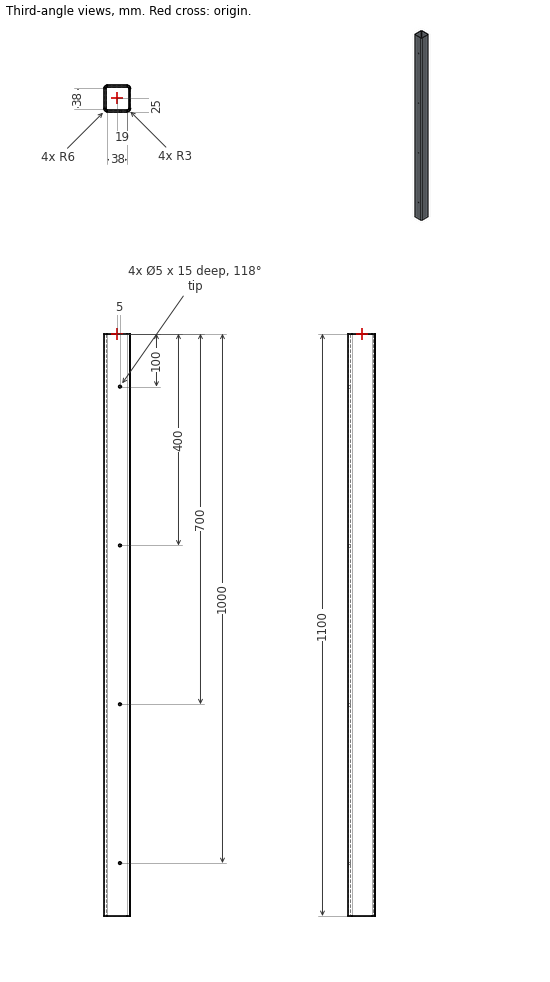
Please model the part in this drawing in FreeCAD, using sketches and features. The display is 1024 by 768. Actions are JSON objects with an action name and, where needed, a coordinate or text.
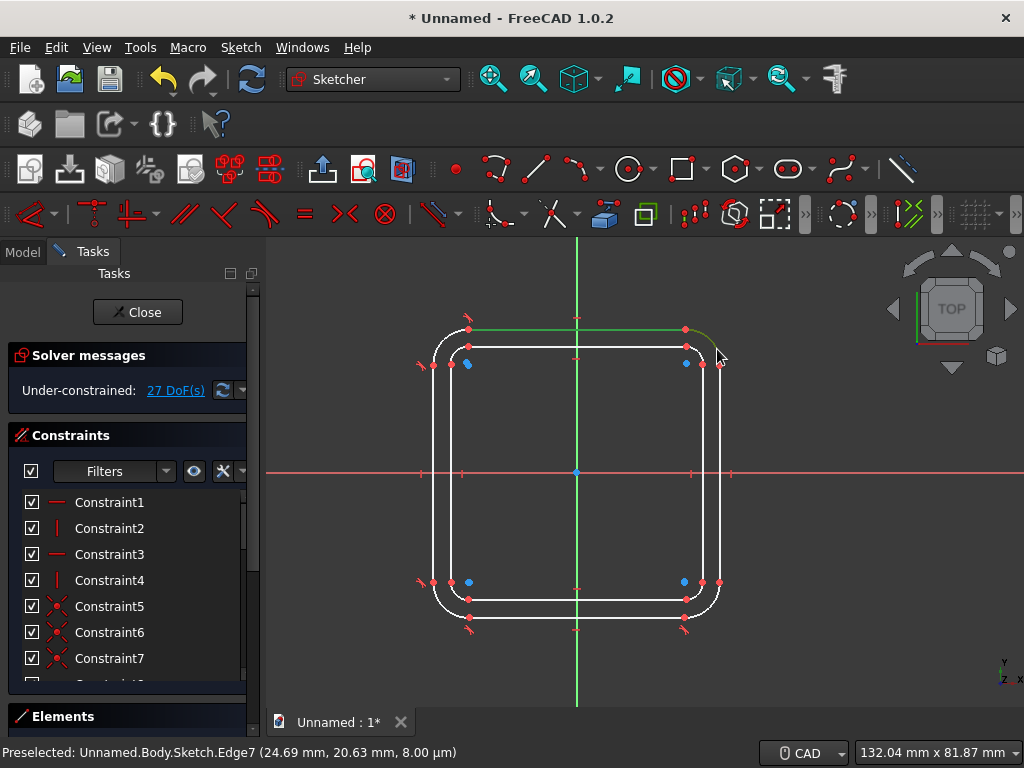
{"action": "key", "text": "t"}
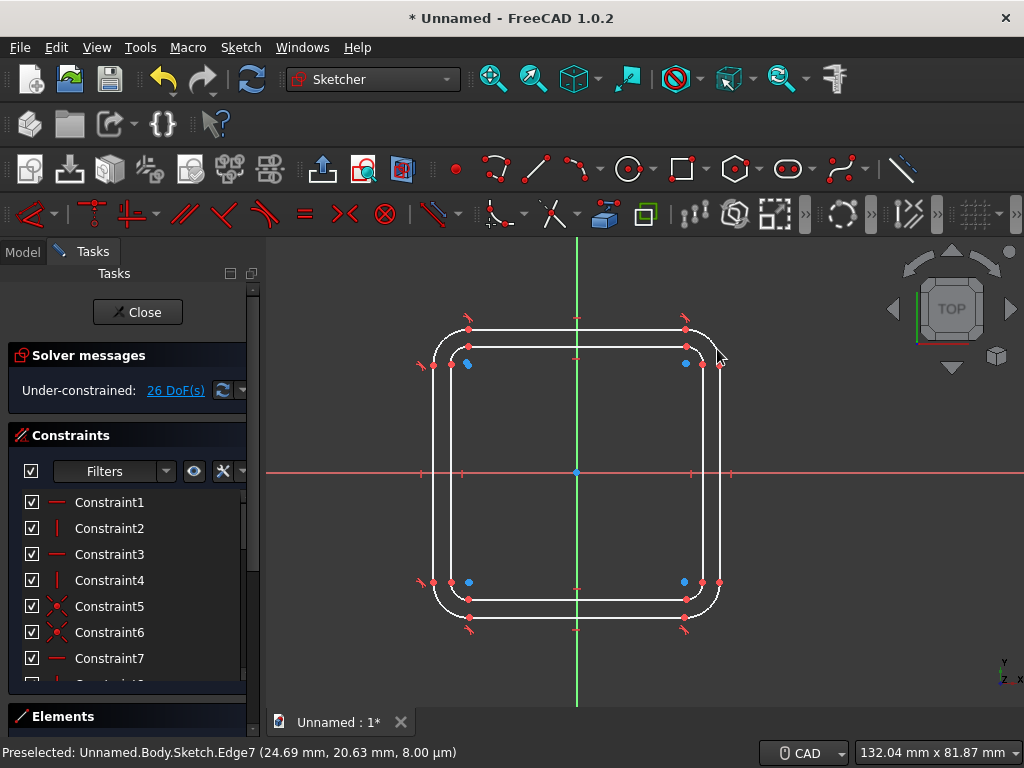
{"action": "left_click", "coordinate": [720, 430]}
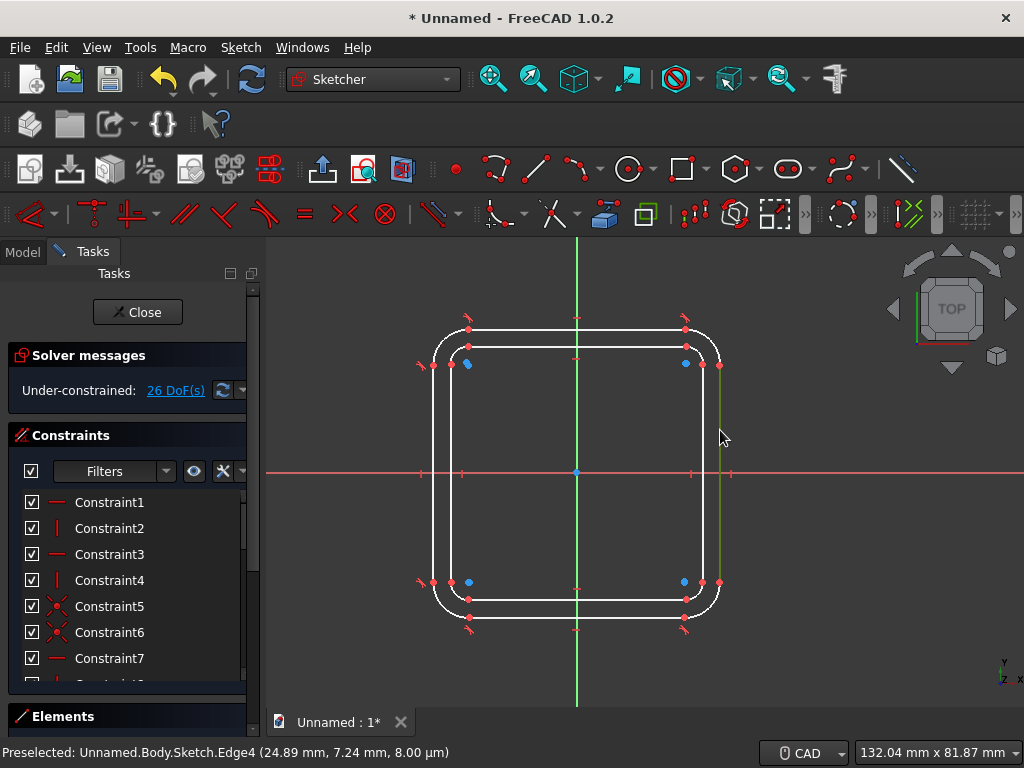
{"action": "left_click", "coordinate": [716, 349]}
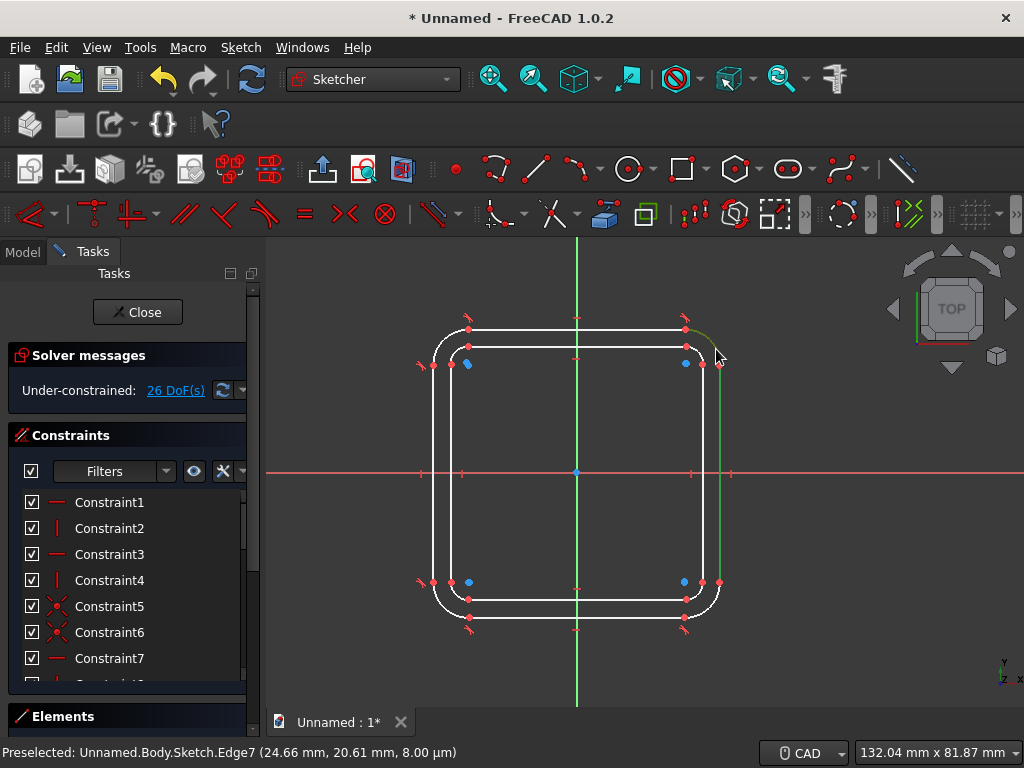
{"action": "key", "text": "t"}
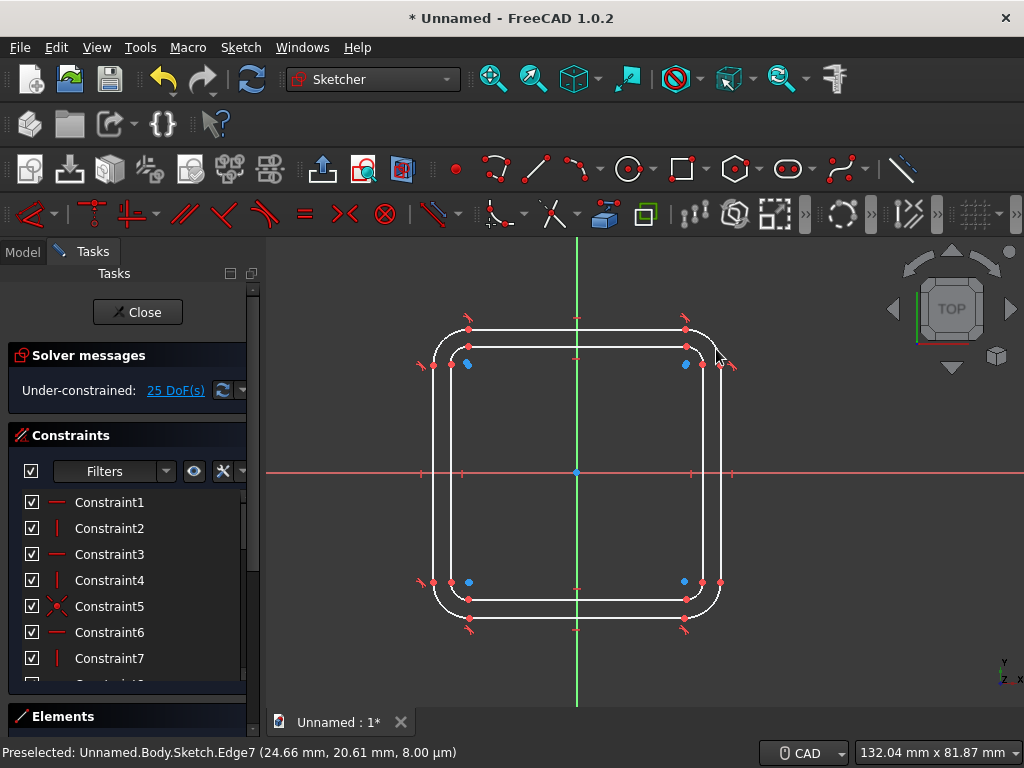
{"action": "left_click", "coordinate": [721, 430]}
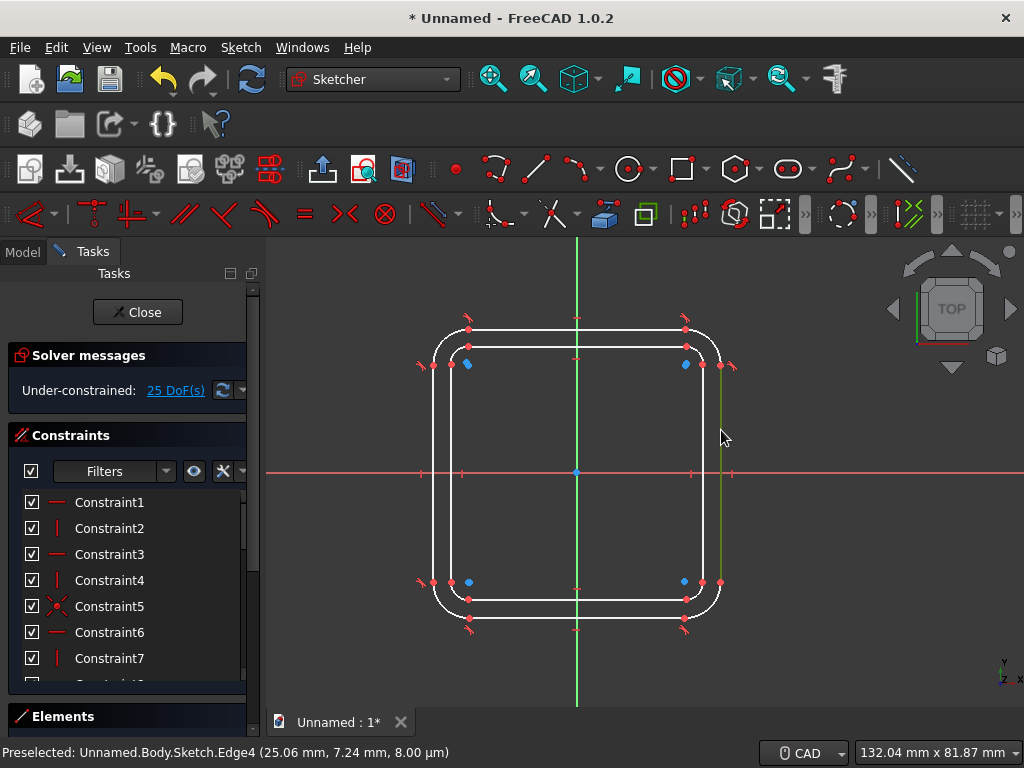
{"action": "left_click", "coordinate": [701, 614]}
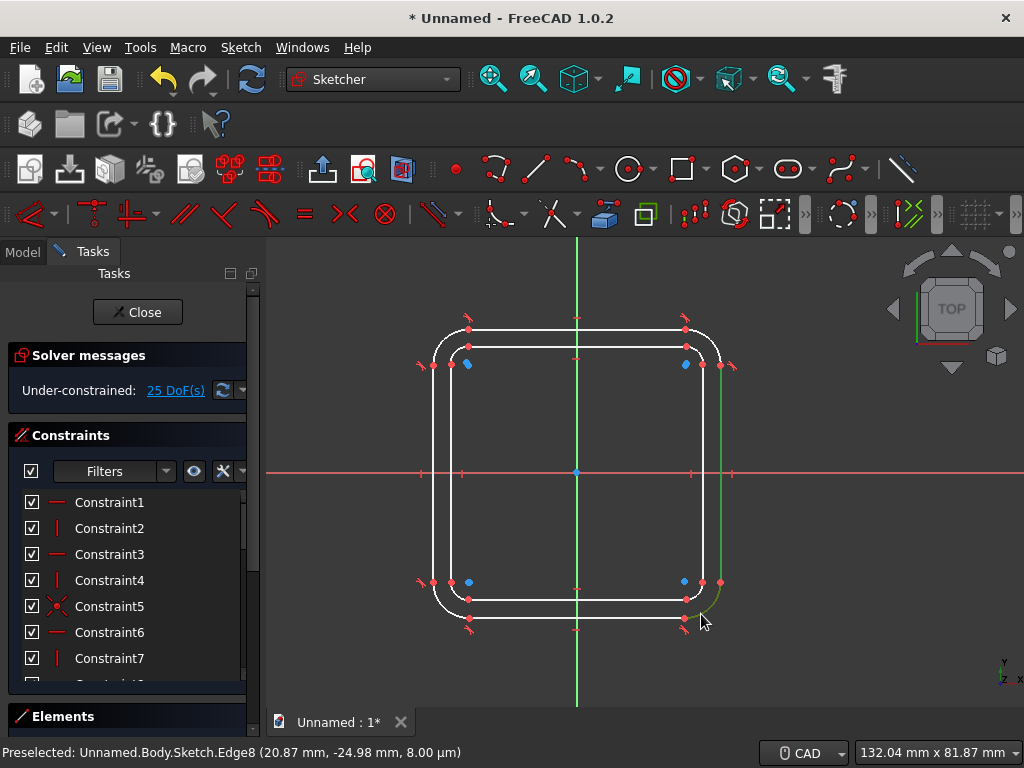
{"action": "key", "text": "t"}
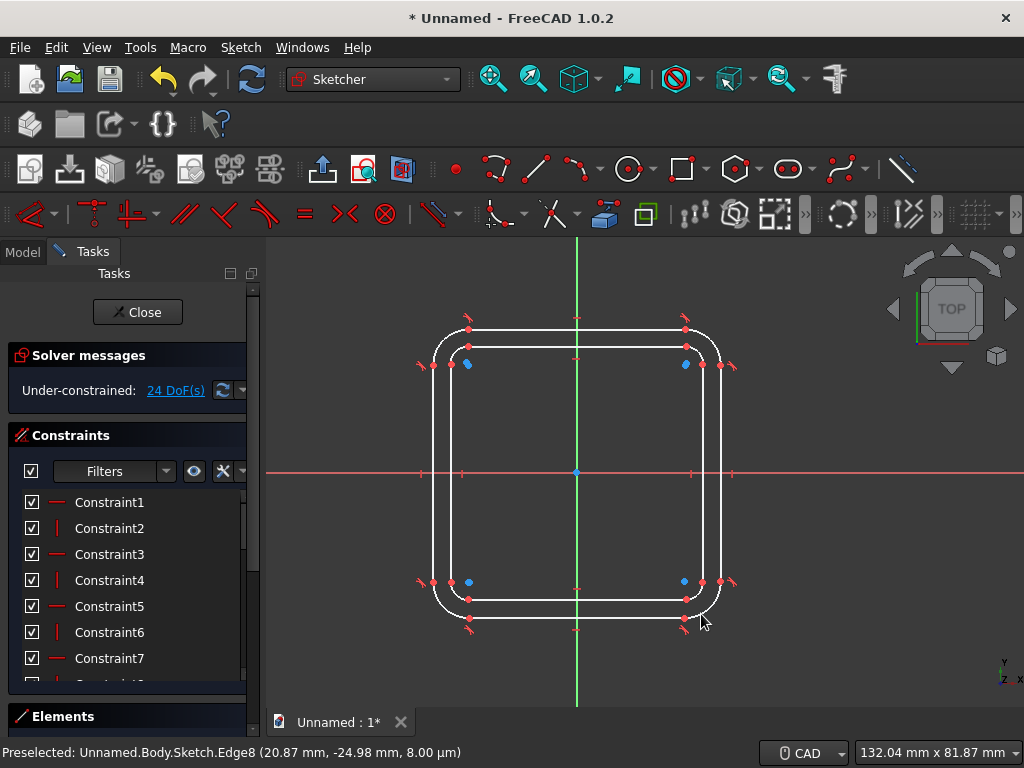
{"action": "left_click", "coordinate": [533, 600]}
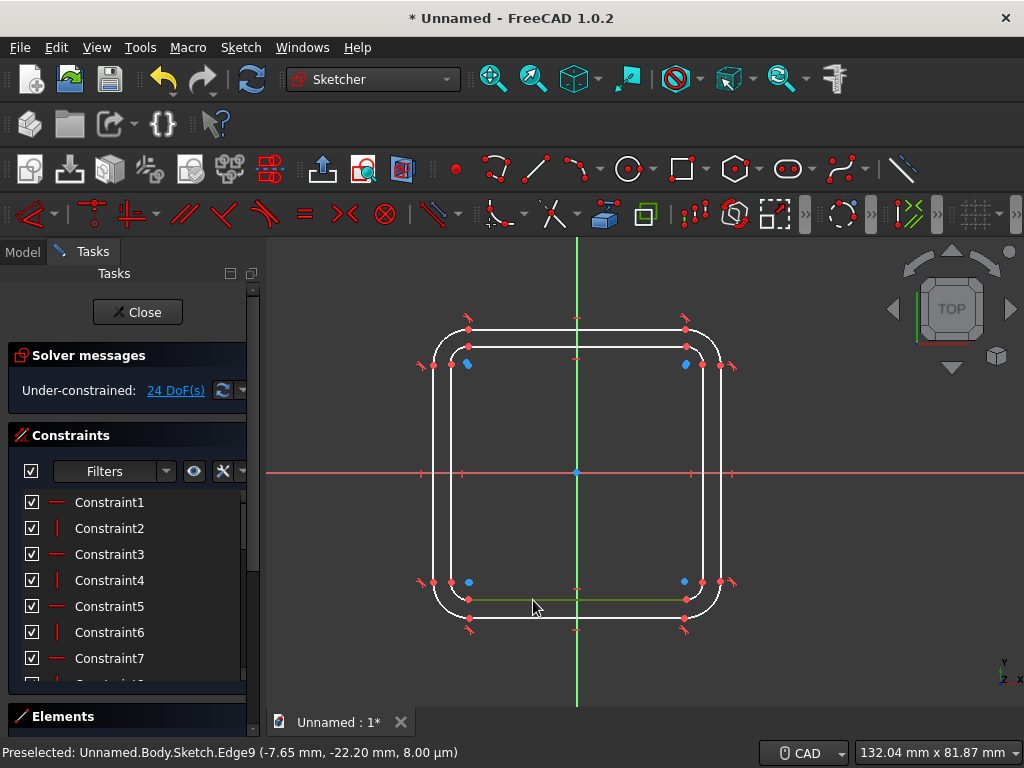
{"action": "left_click", "coordinate": [698, 595]}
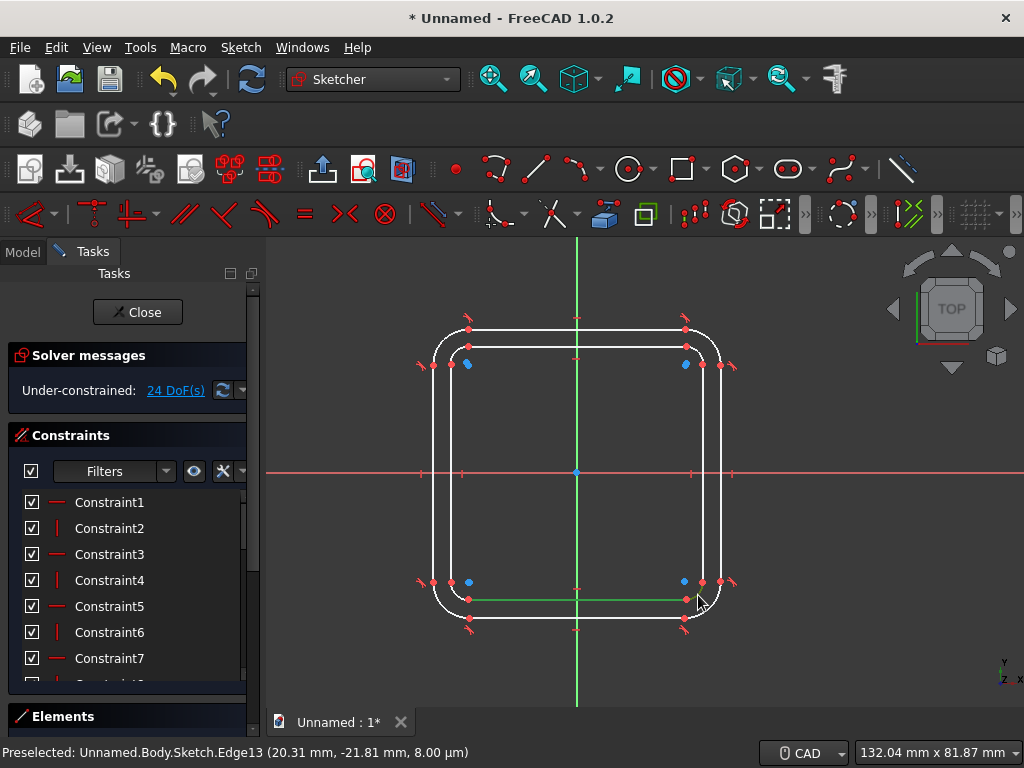
{"action": "key", "text": "t"}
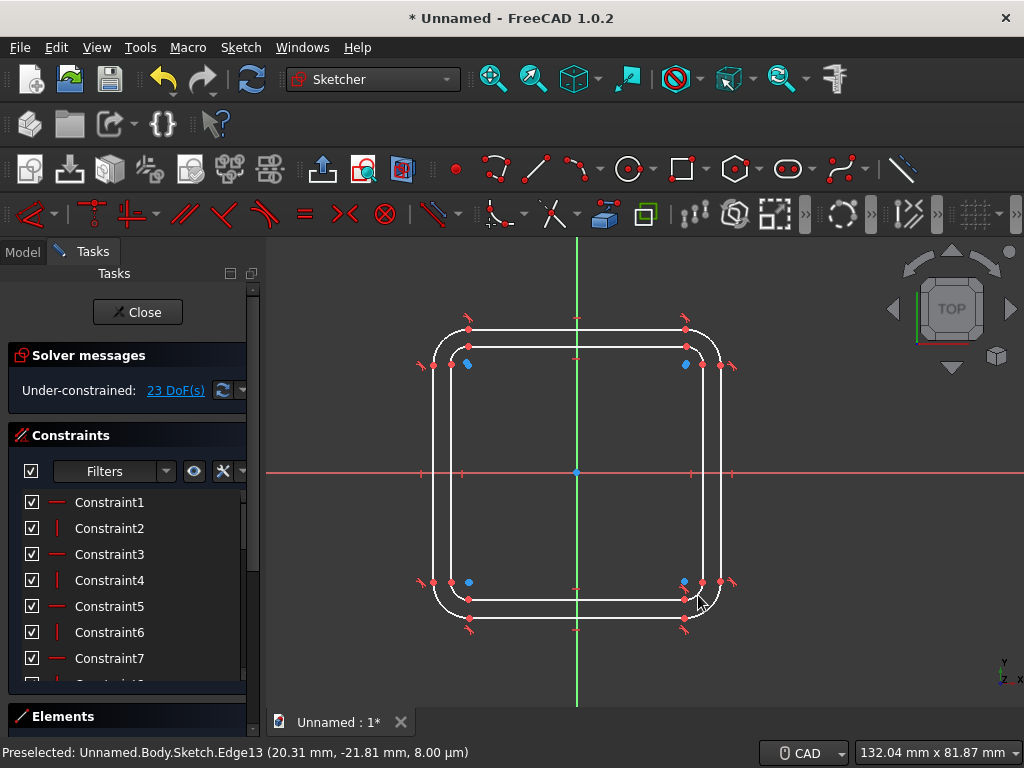
{"action": "left_click", "coordinate": [533, 600]}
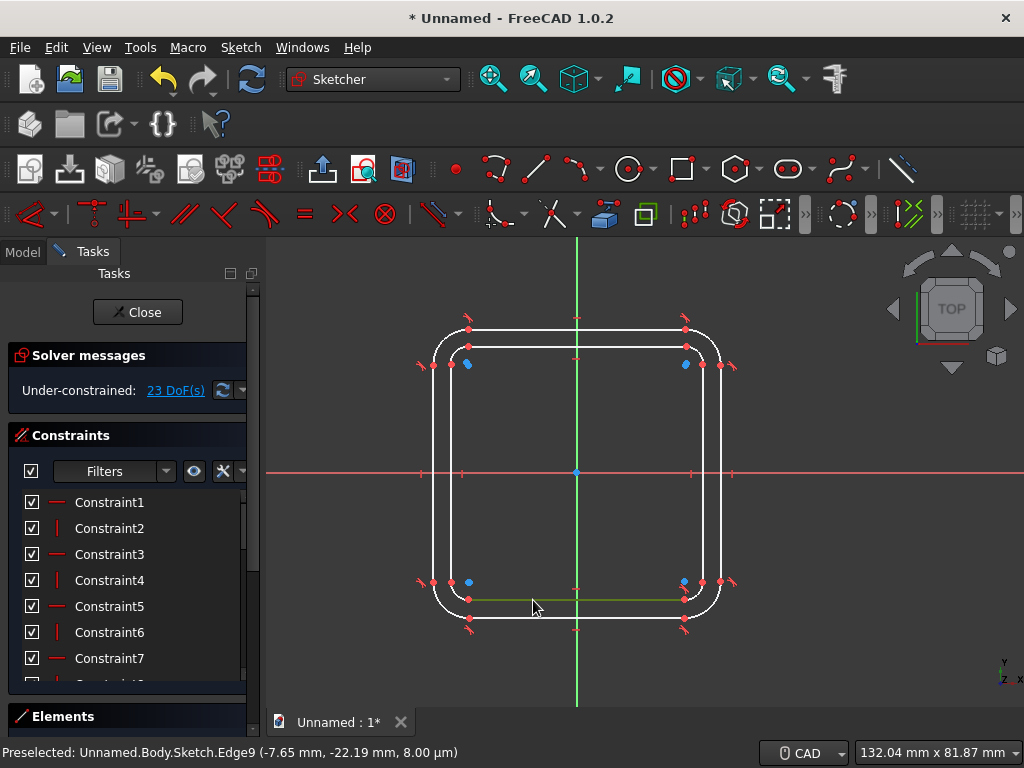
{"action": "left_click", "coordinate": [456, 595]}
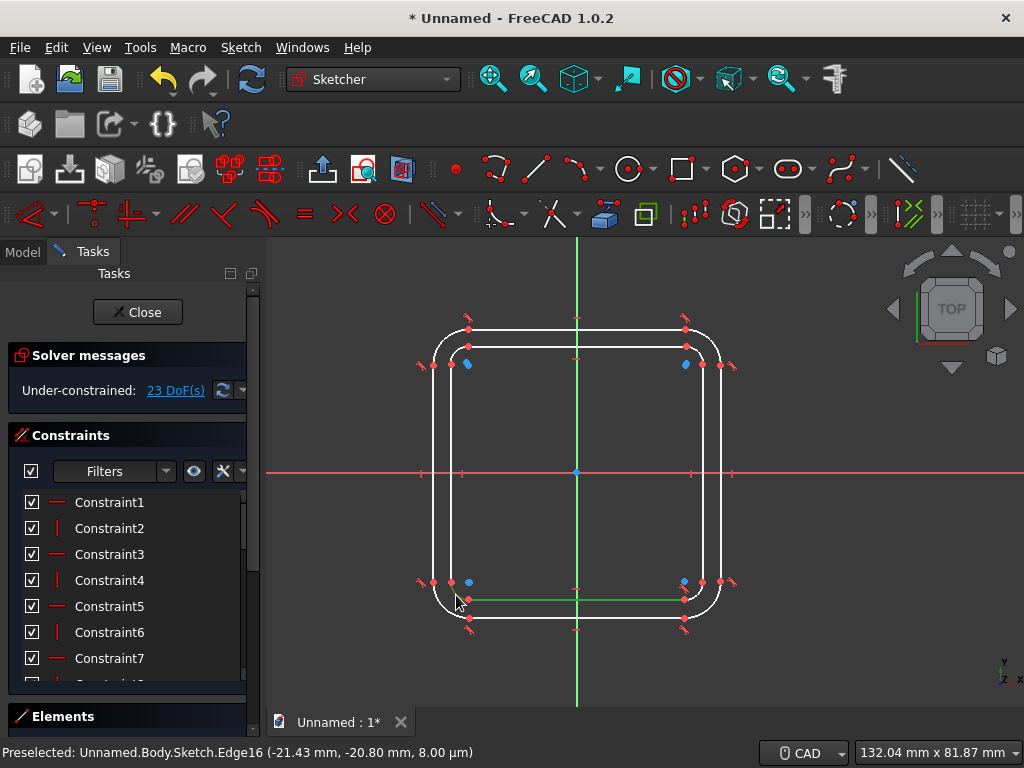
{"action": "key", "text": "t"}